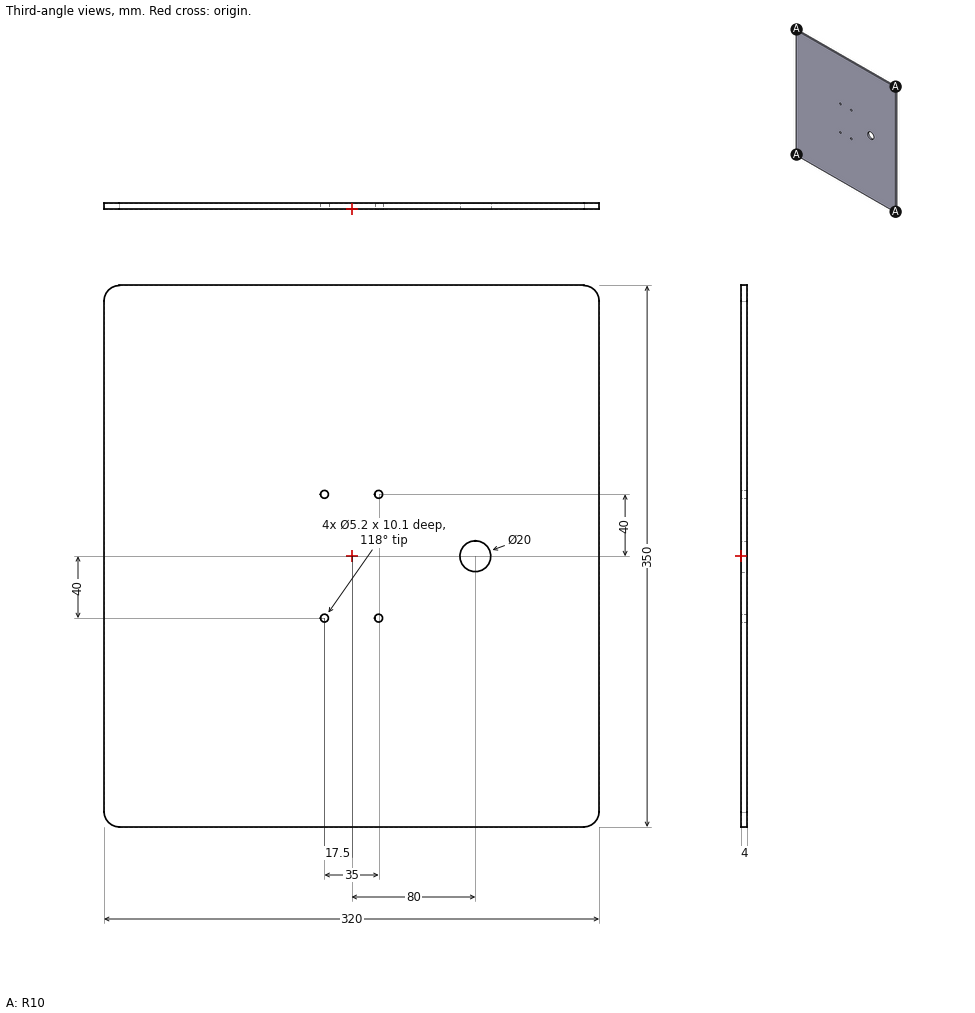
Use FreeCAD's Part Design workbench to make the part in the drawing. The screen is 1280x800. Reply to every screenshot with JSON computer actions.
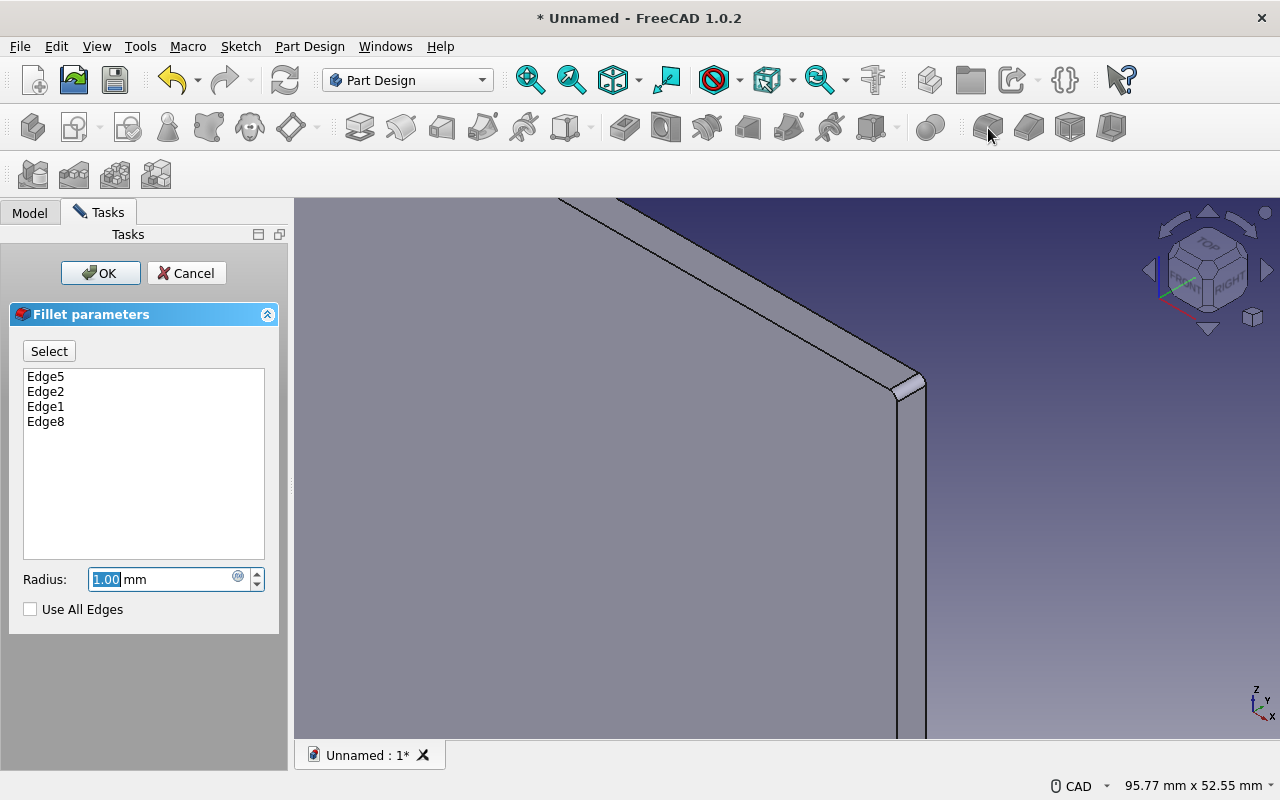
{"action": "type", "text": "10"}
{"action": "key", "text": "Tab"}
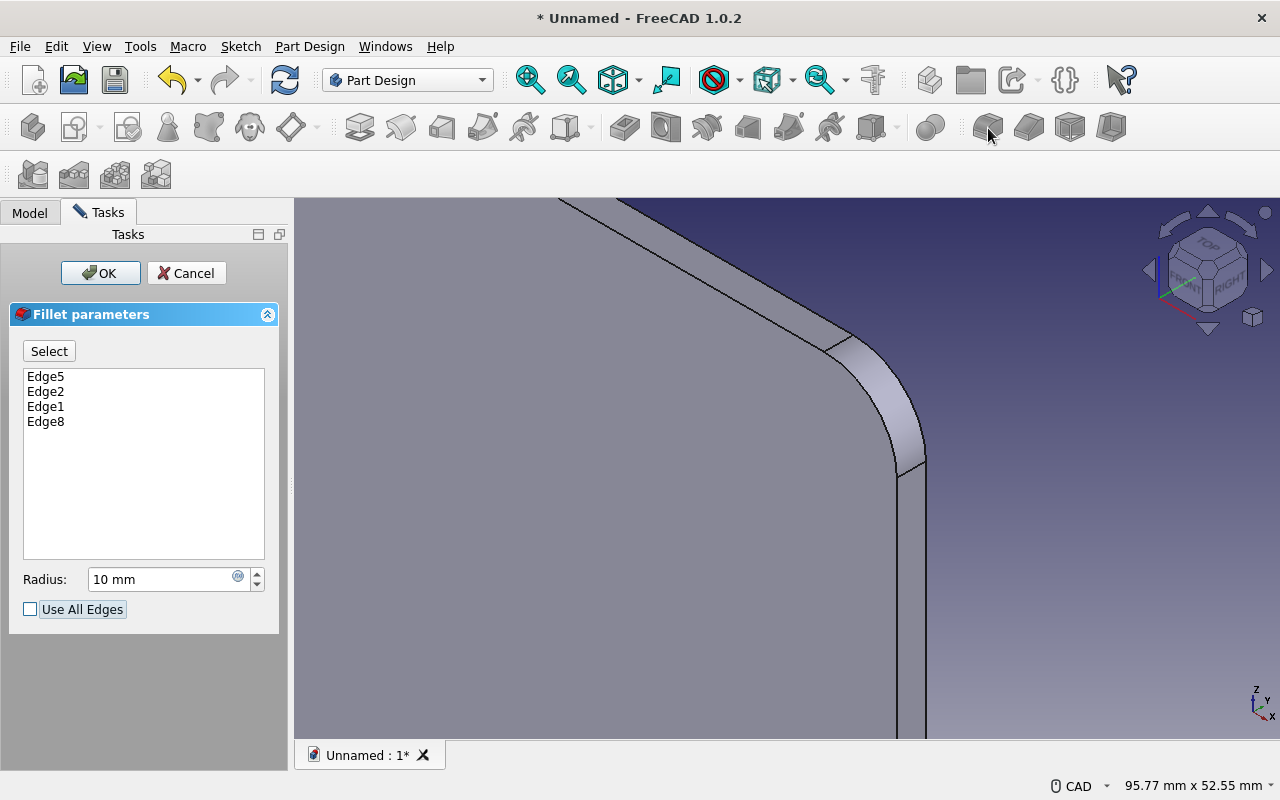
{"action": "left_click", "coordinate": [101, 273]}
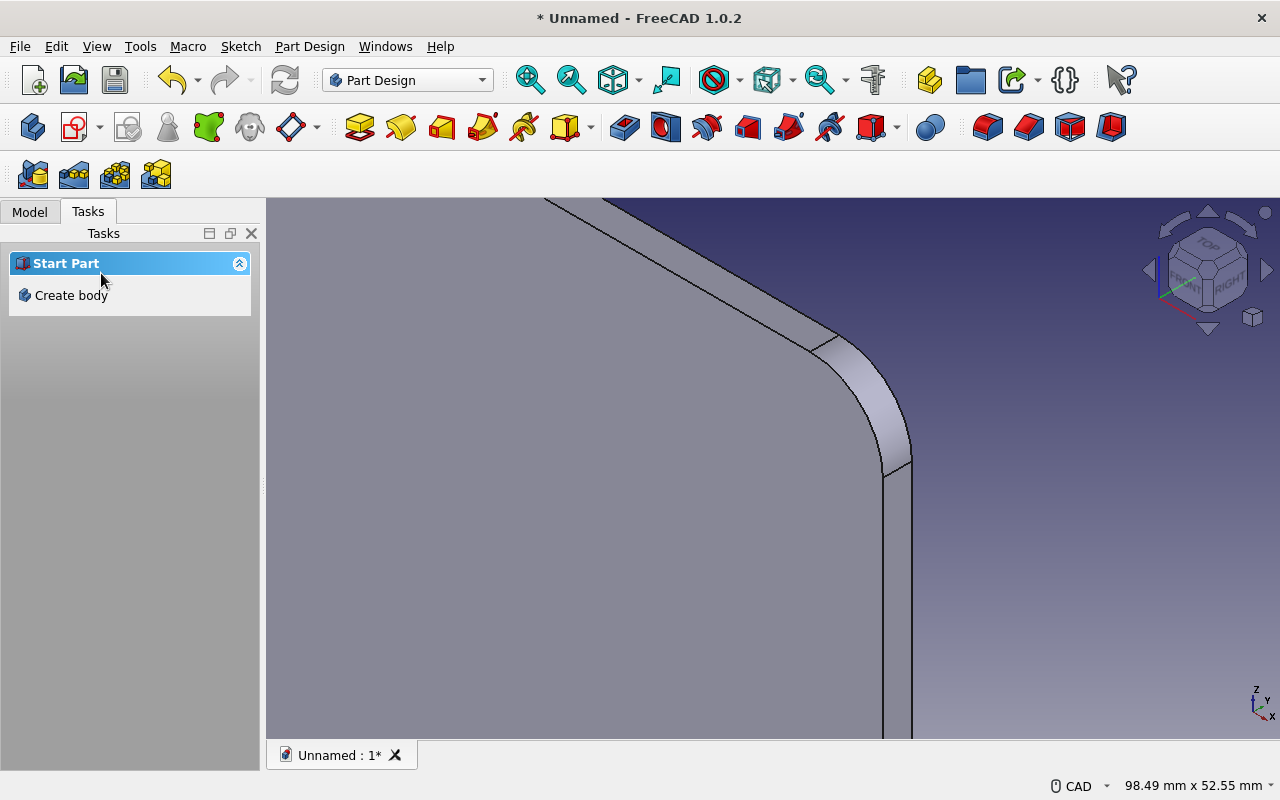
{"action": "left_click", "coordinate": [531, 80]}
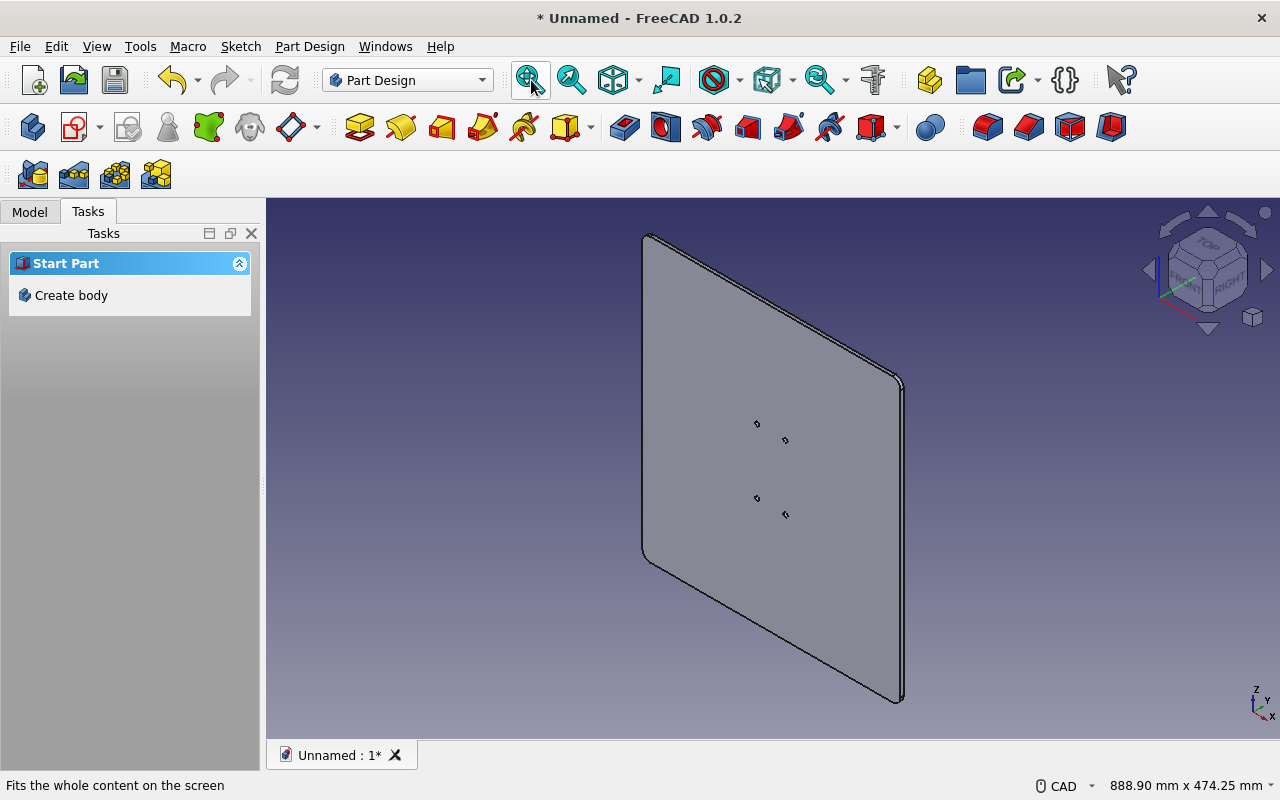
{"action": "key", "text": "4"}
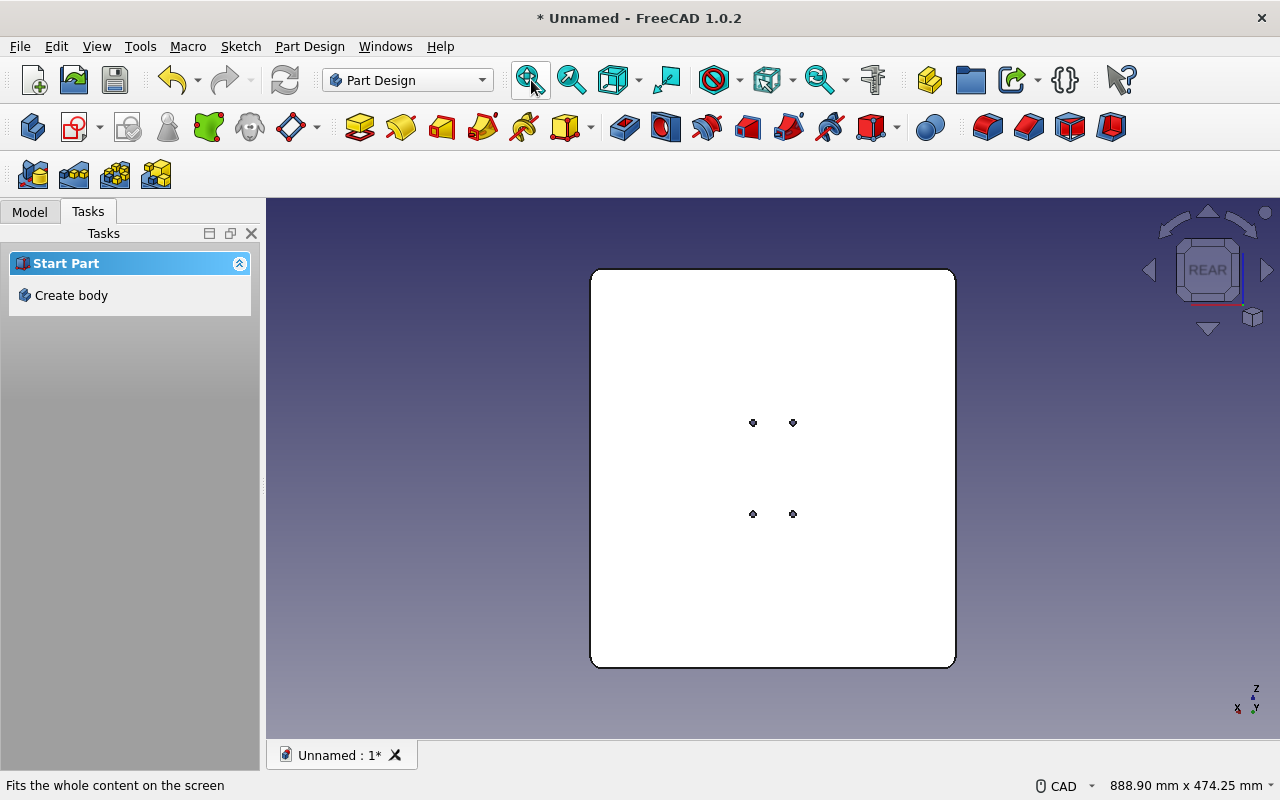
{"action": "left_click", "coordinate": [669, 353]}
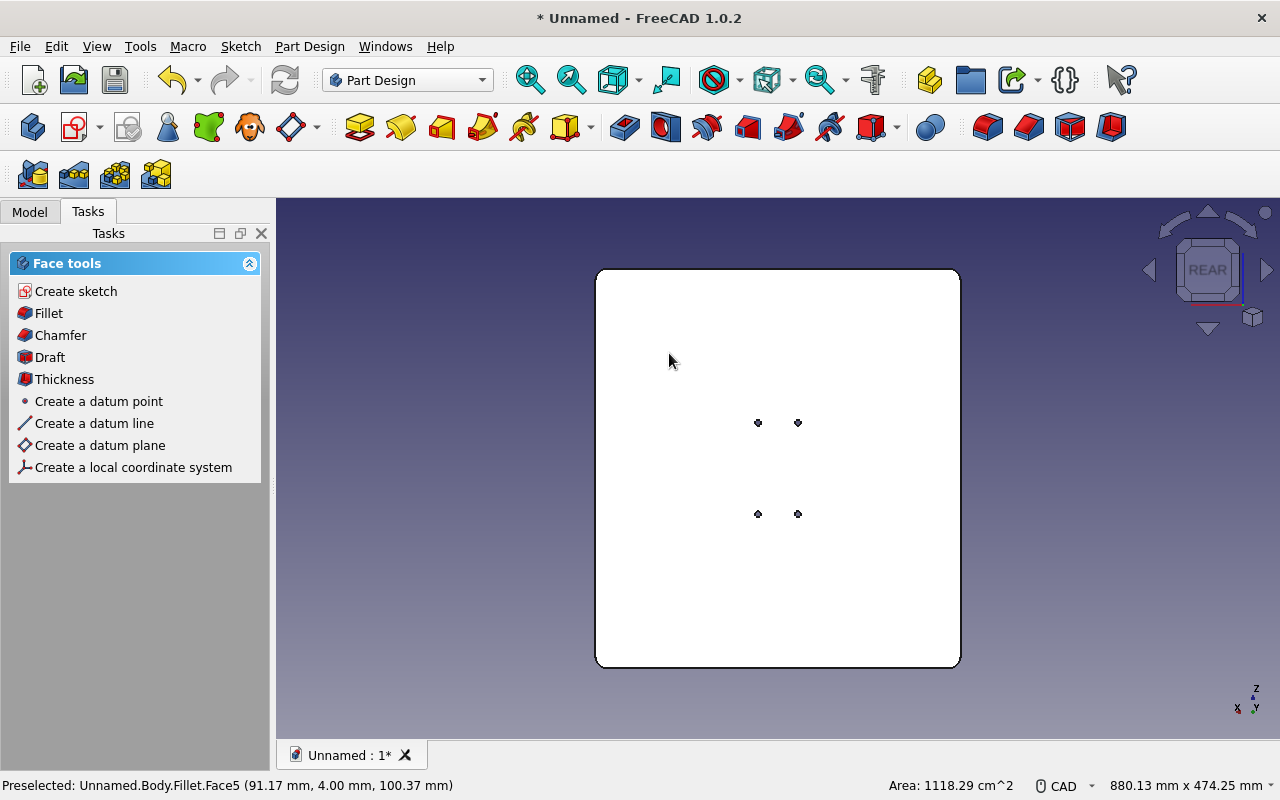
{"action": "left_click", "coordinate": [74, 128]}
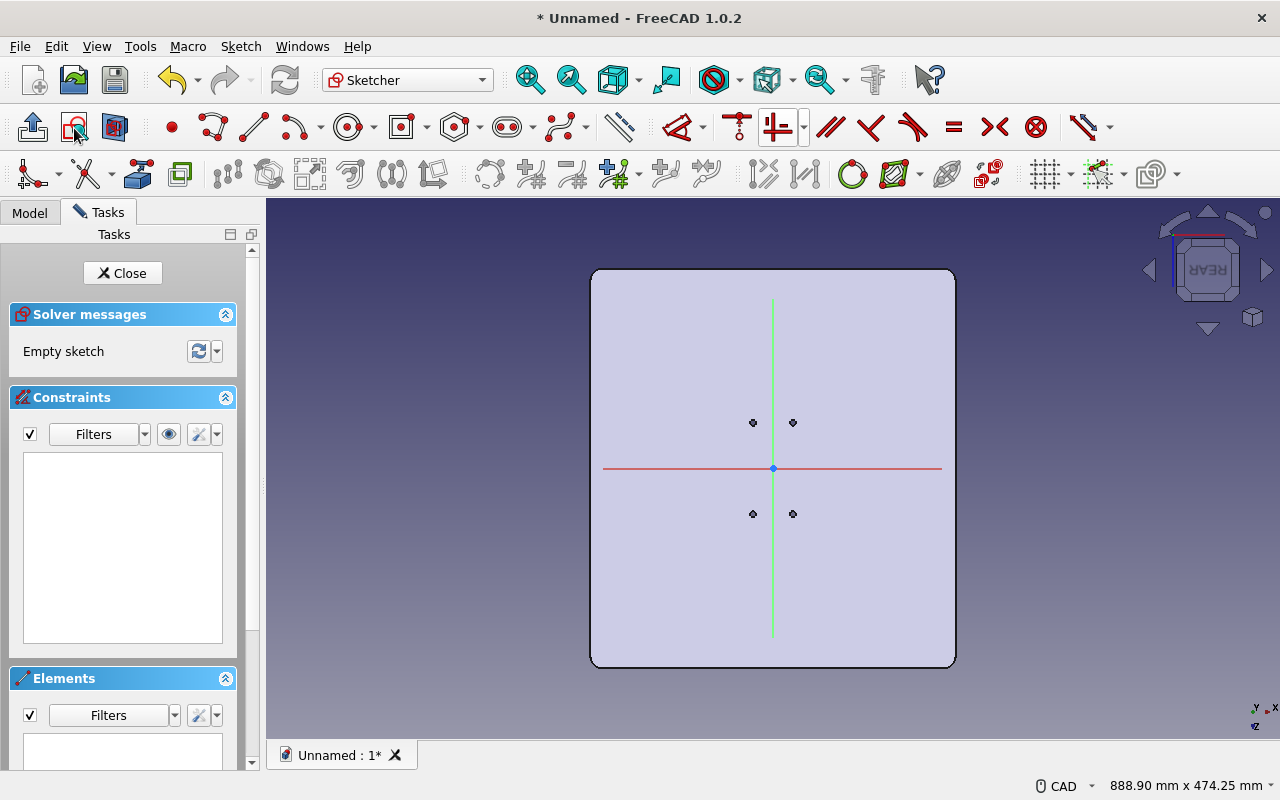
{"action": "scroll", "coordinate": [875, 468], "scroll_direction": "up", "scroll_amount": 14}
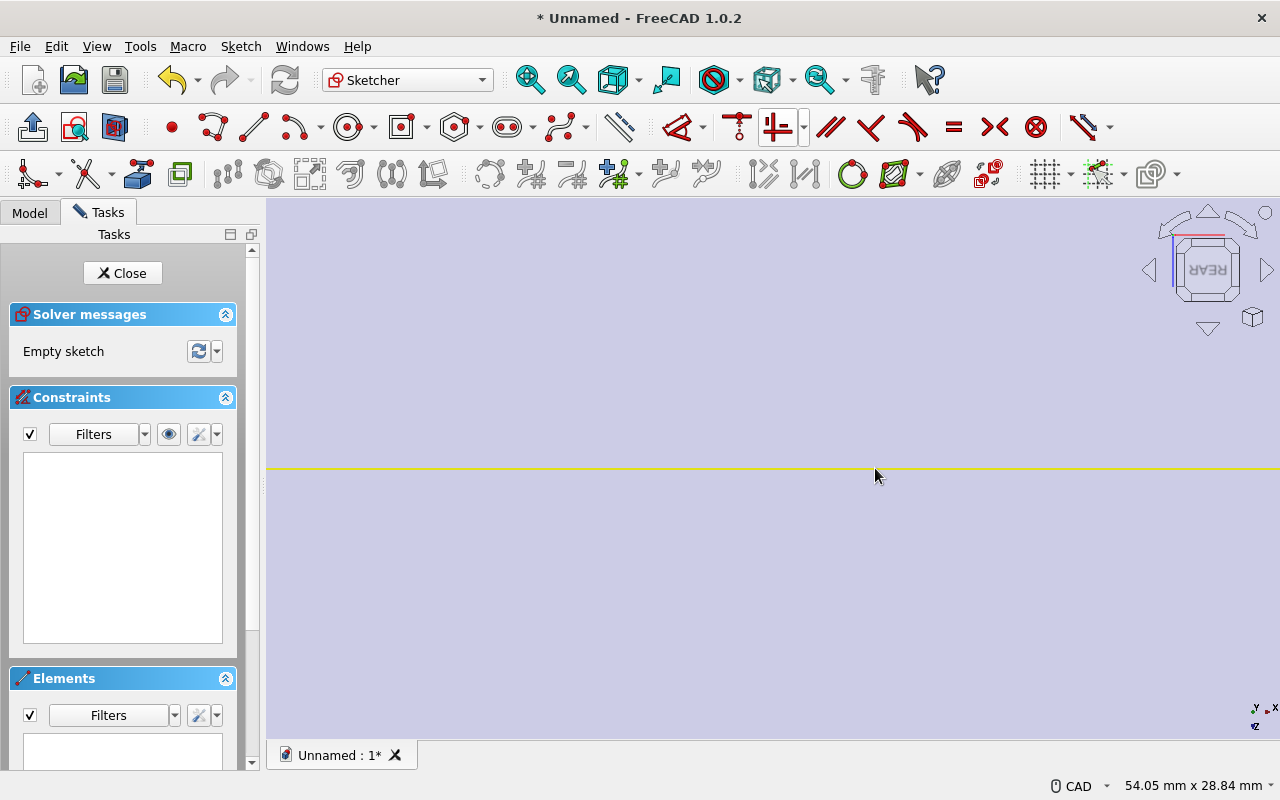
{"action": "left_click", "coordinate": [348, 128]}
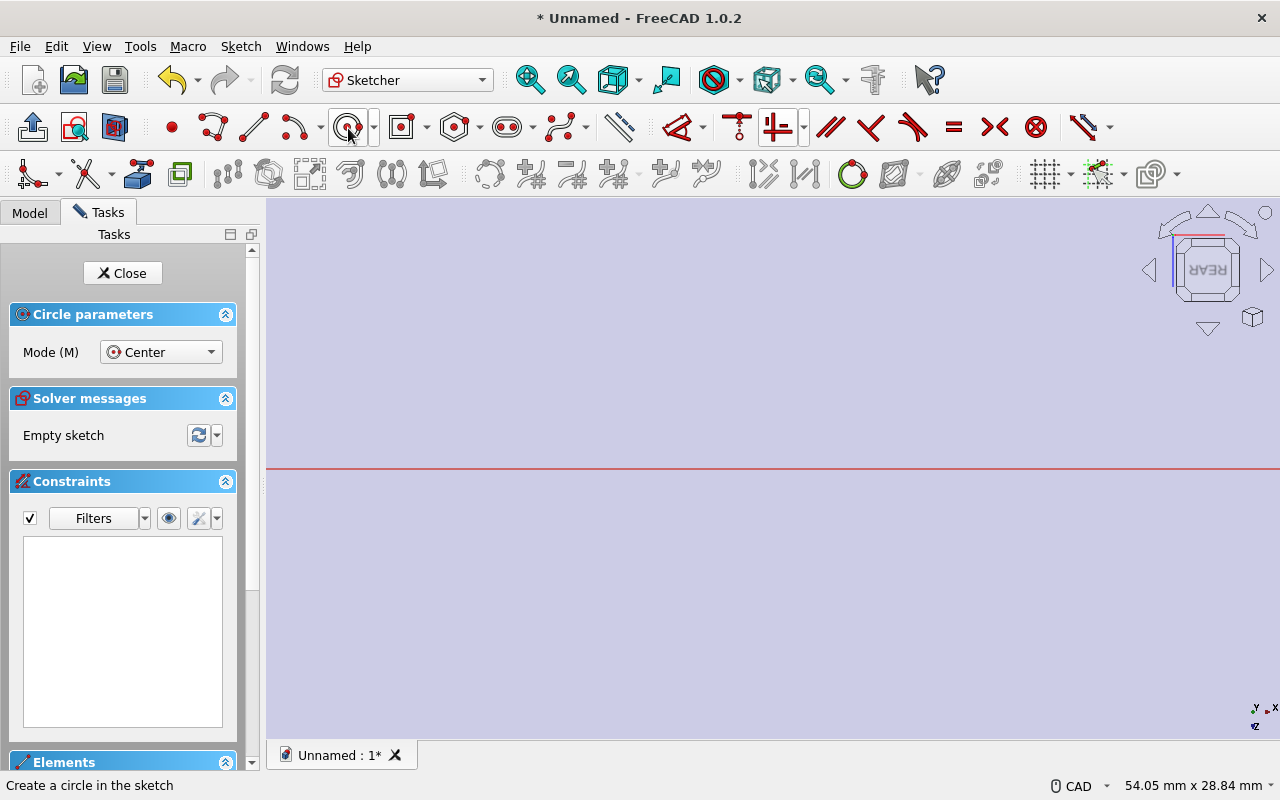
{"action": "left_click", "coordinate": [689, 468]}
{"action": "left_click", "coordinate": [822, 336]}
{"action": "key", "text": "Escape"}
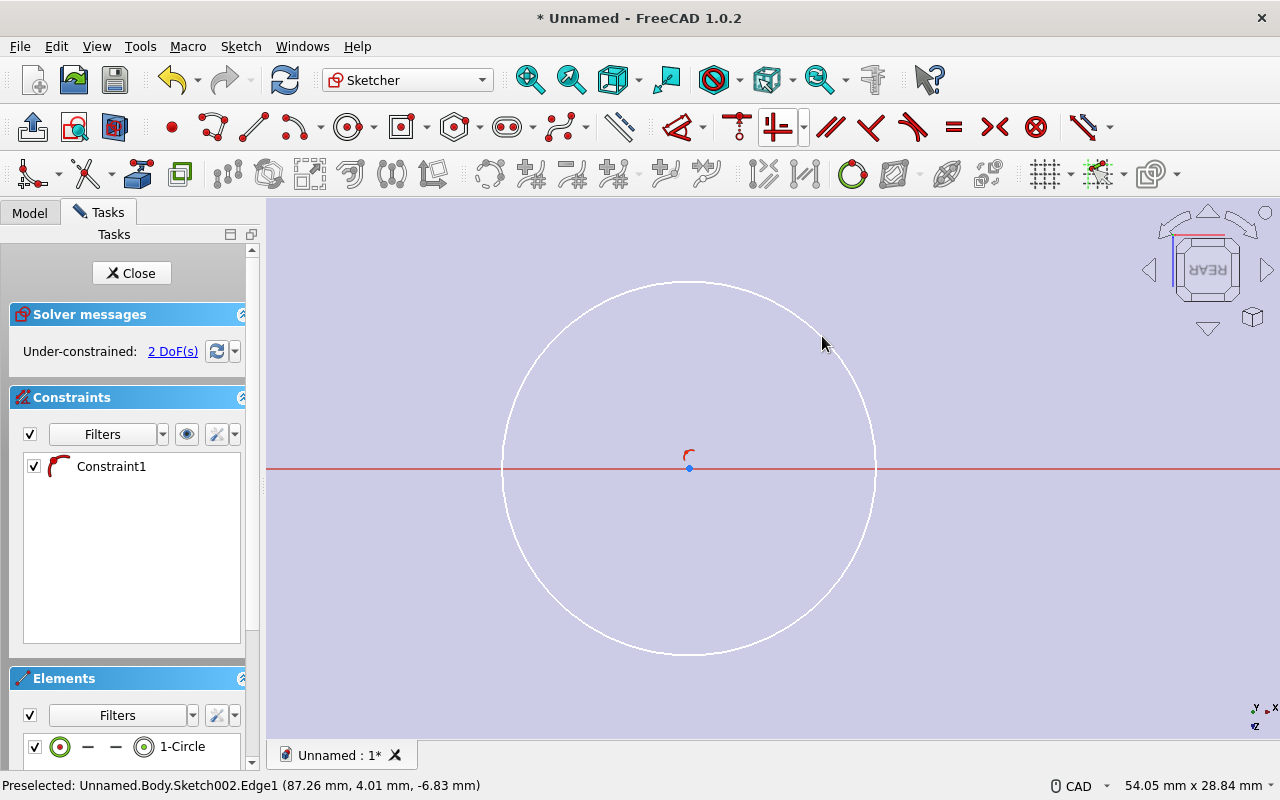
{"action": "key", "text": "d"}